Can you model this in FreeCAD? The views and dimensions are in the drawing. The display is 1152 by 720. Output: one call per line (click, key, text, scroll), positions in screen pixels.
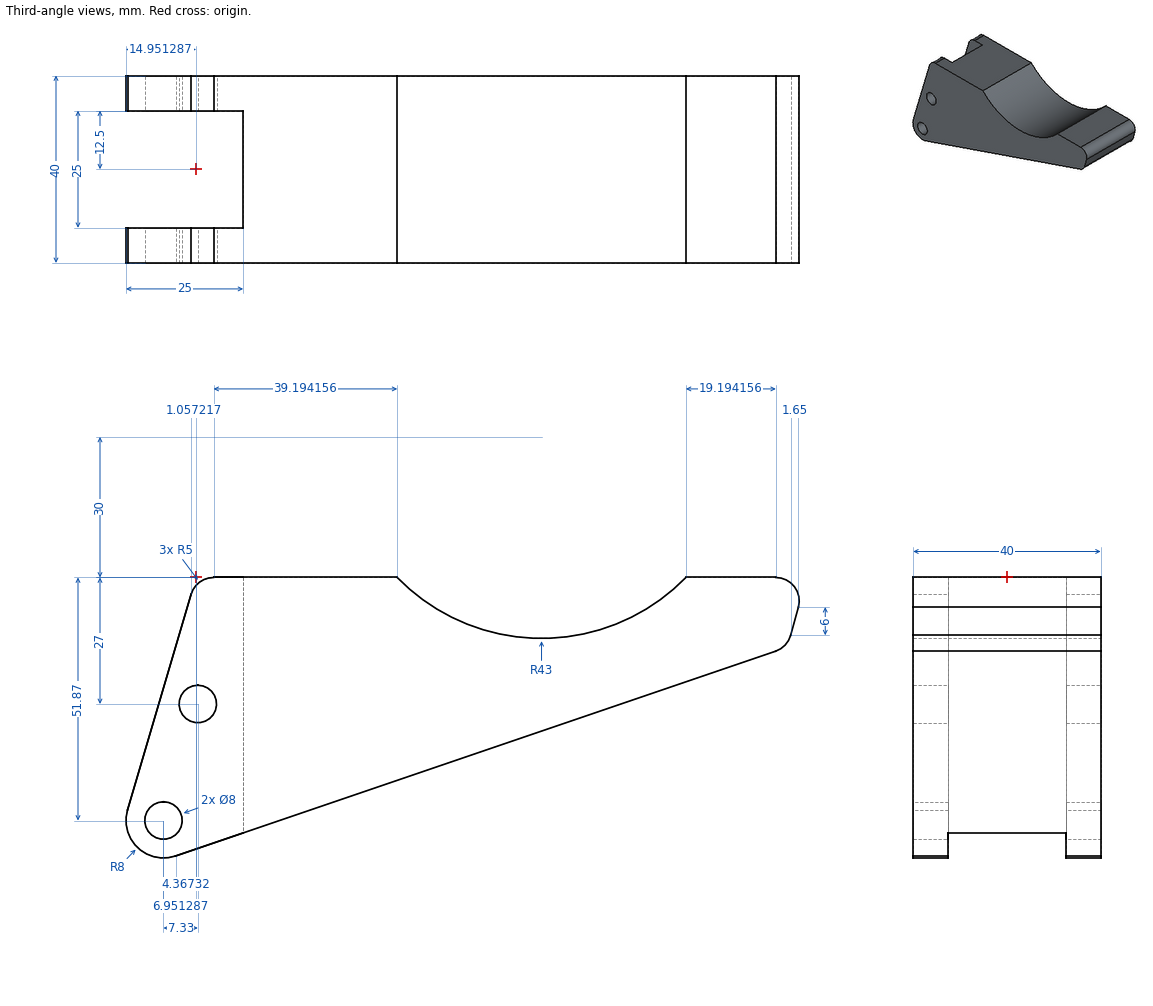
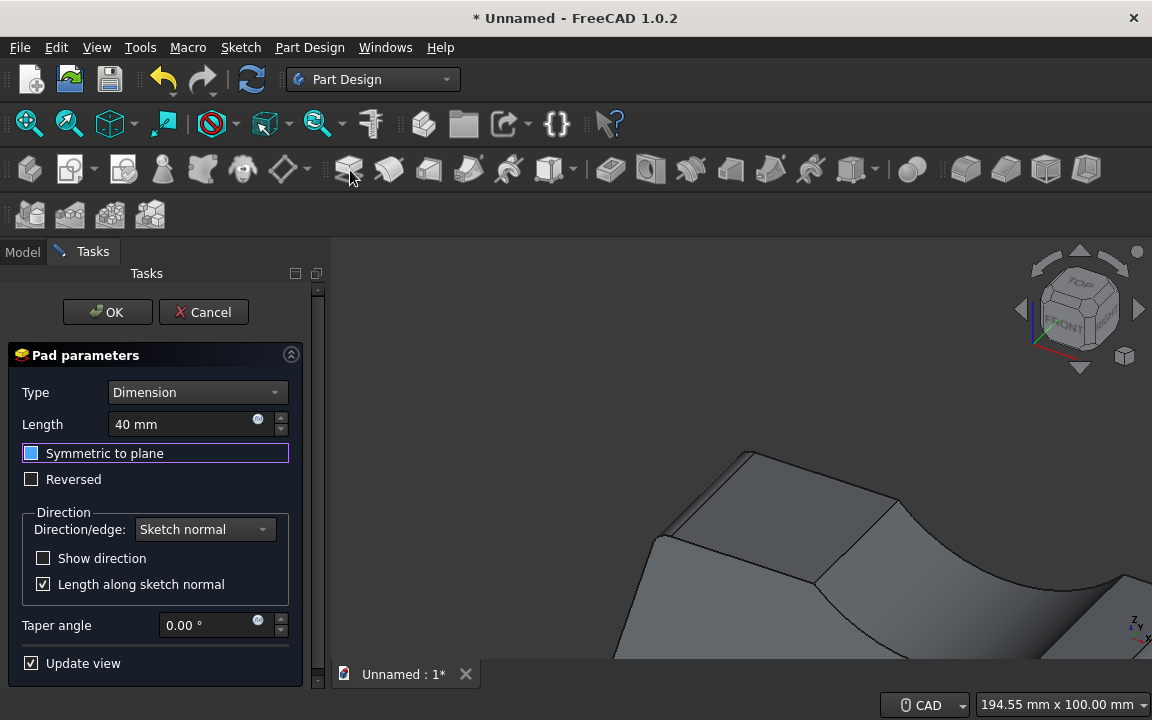
click(30, 453)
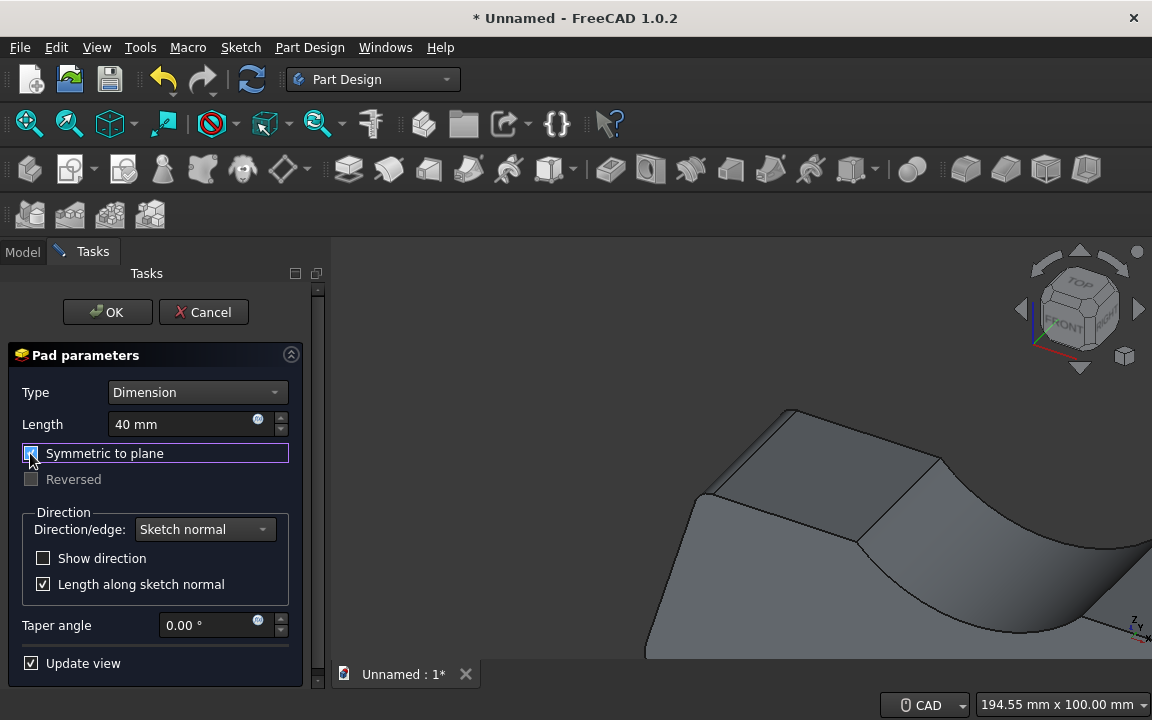
click(108, 312)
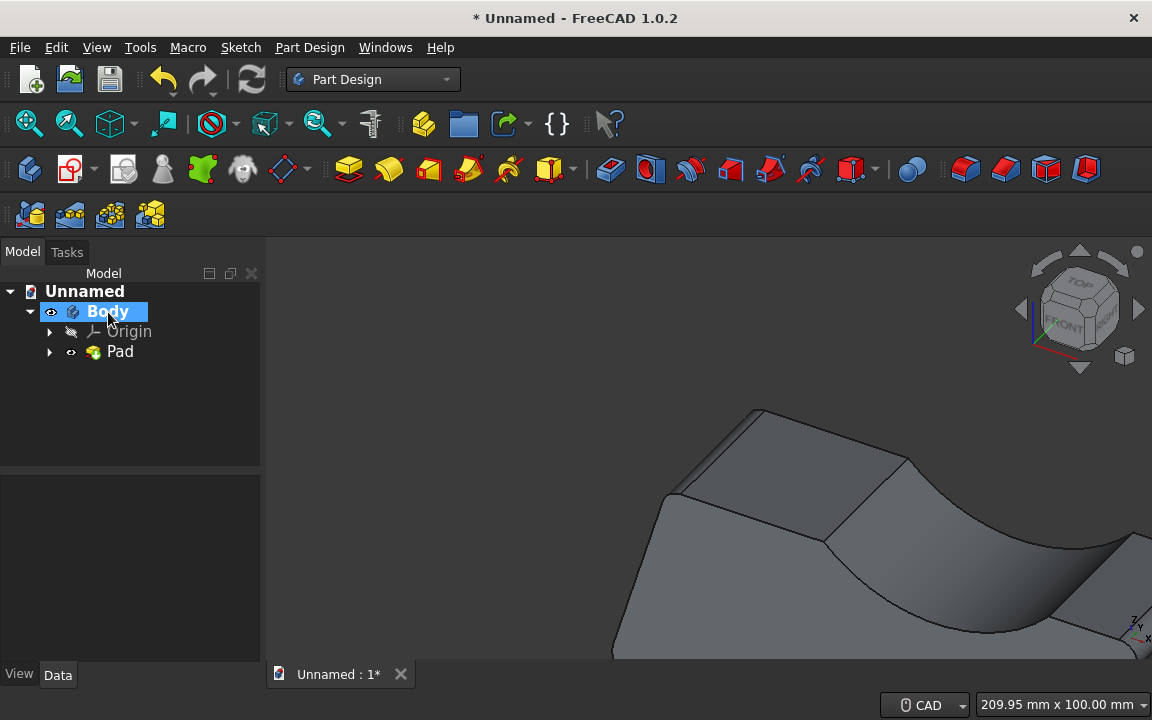
click(30, 124)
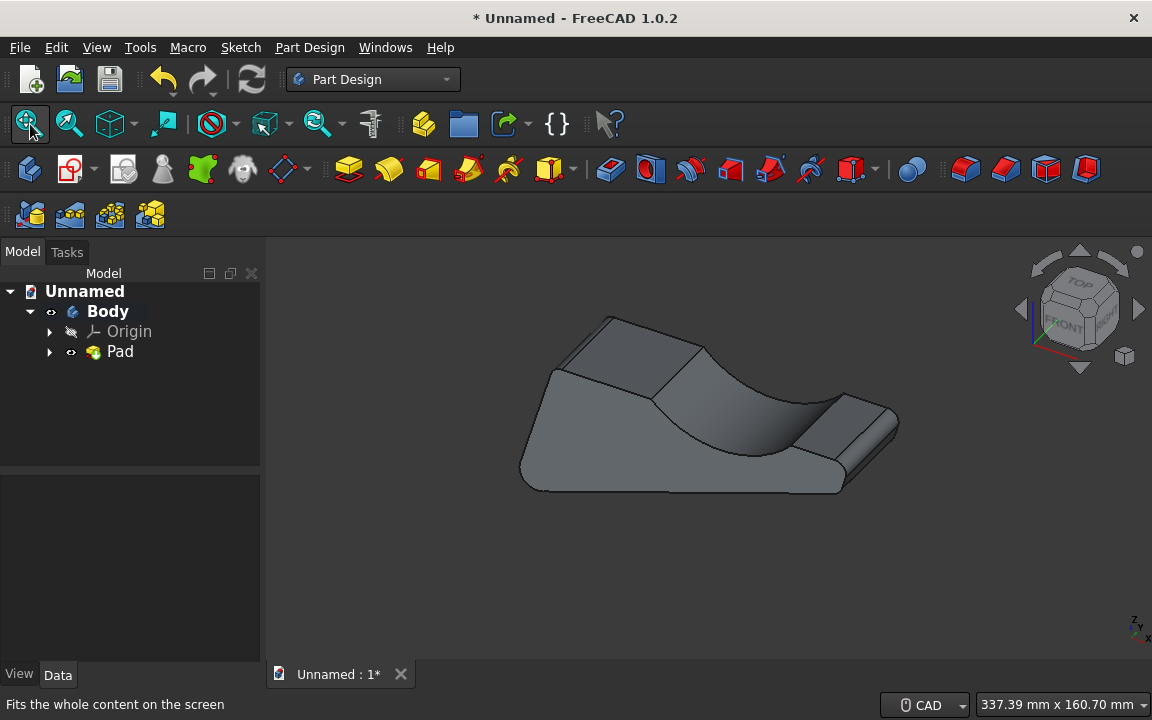
click(70, 170)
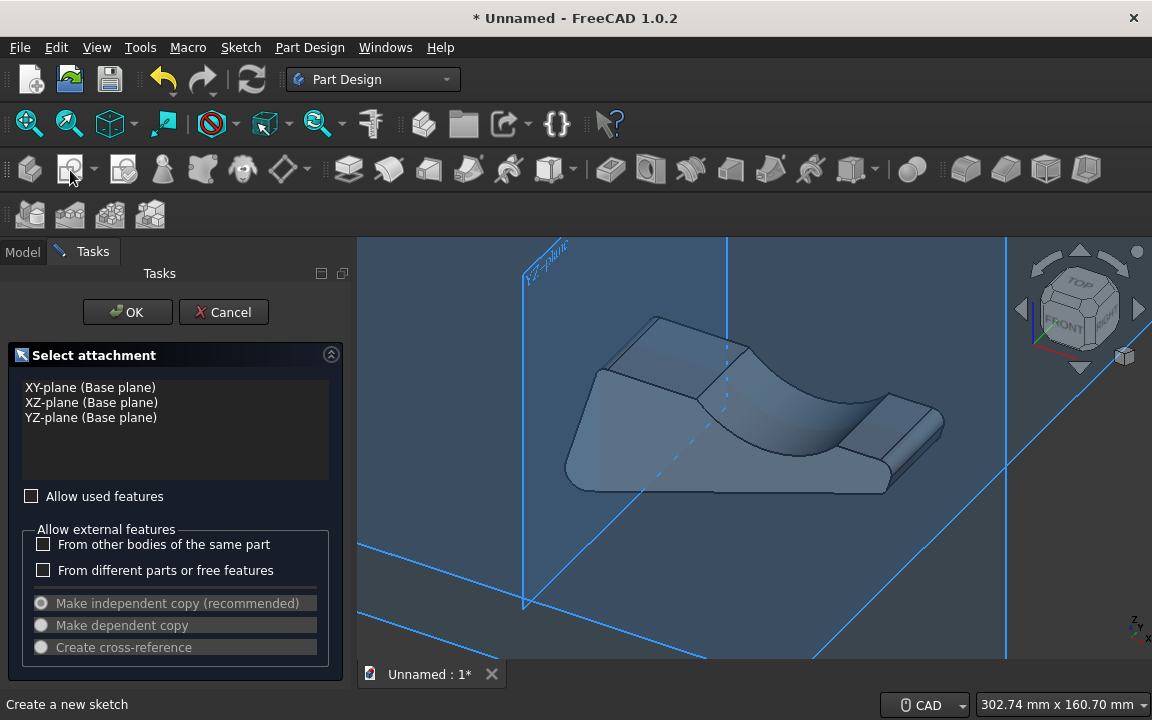
click(82, 402)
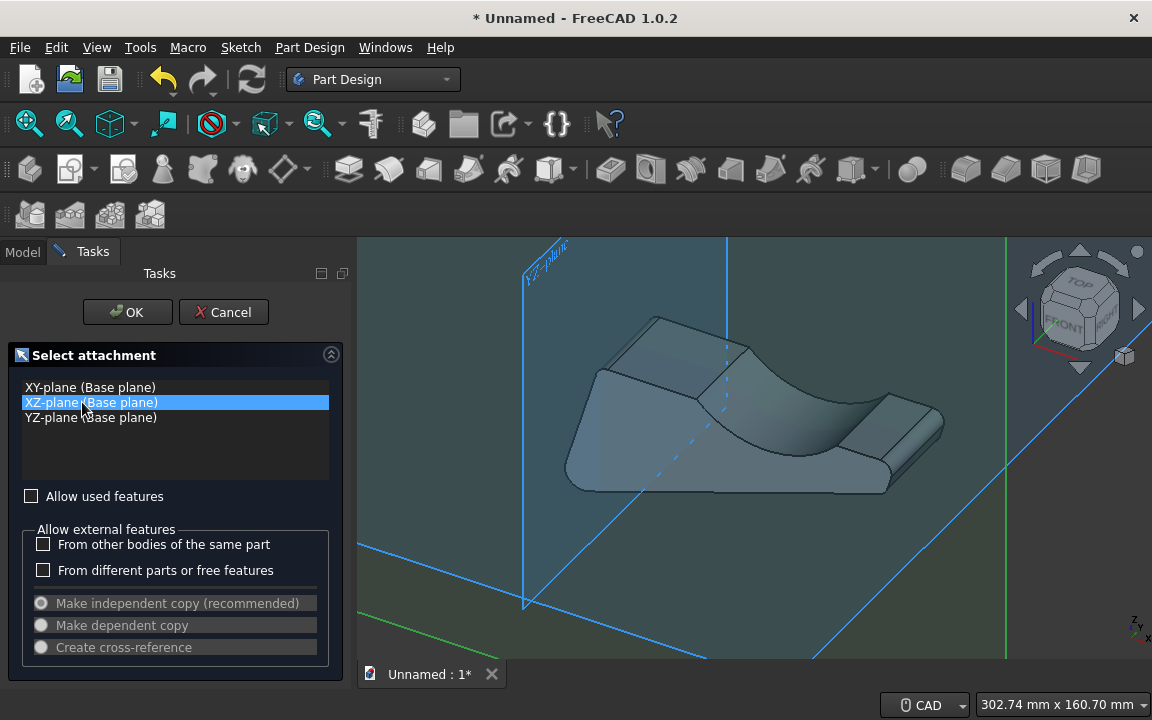
click(128, 312)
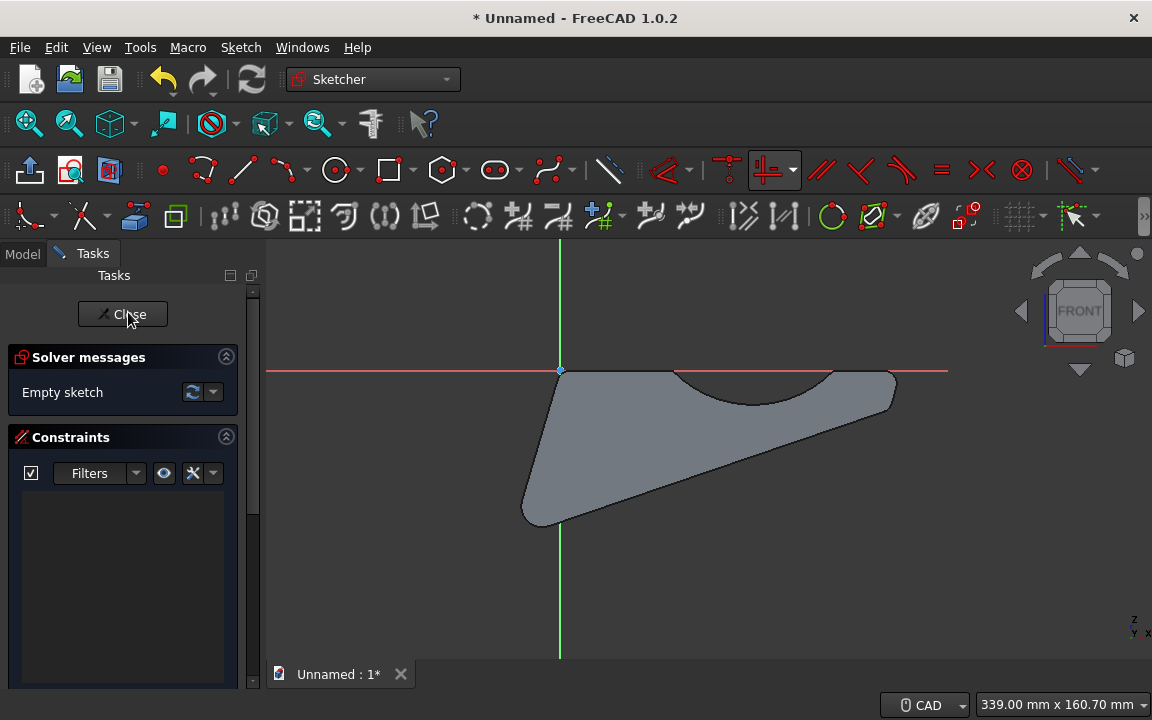
click(110, 170)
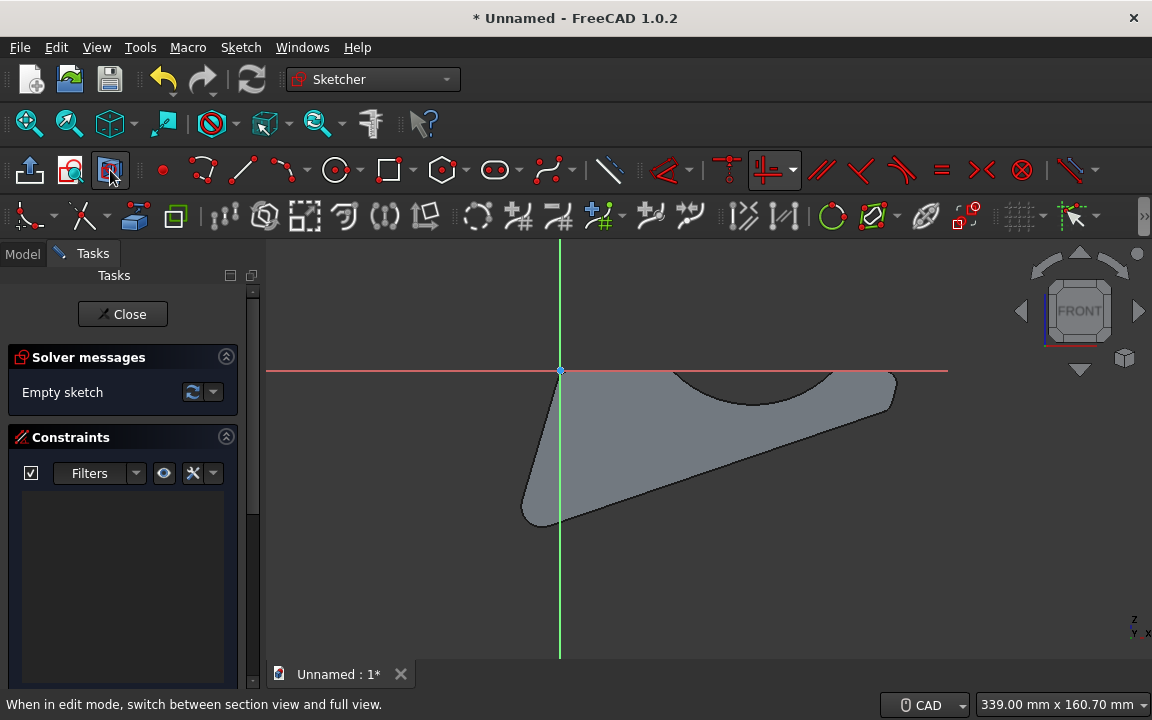
scroll(444, 438, up, 3)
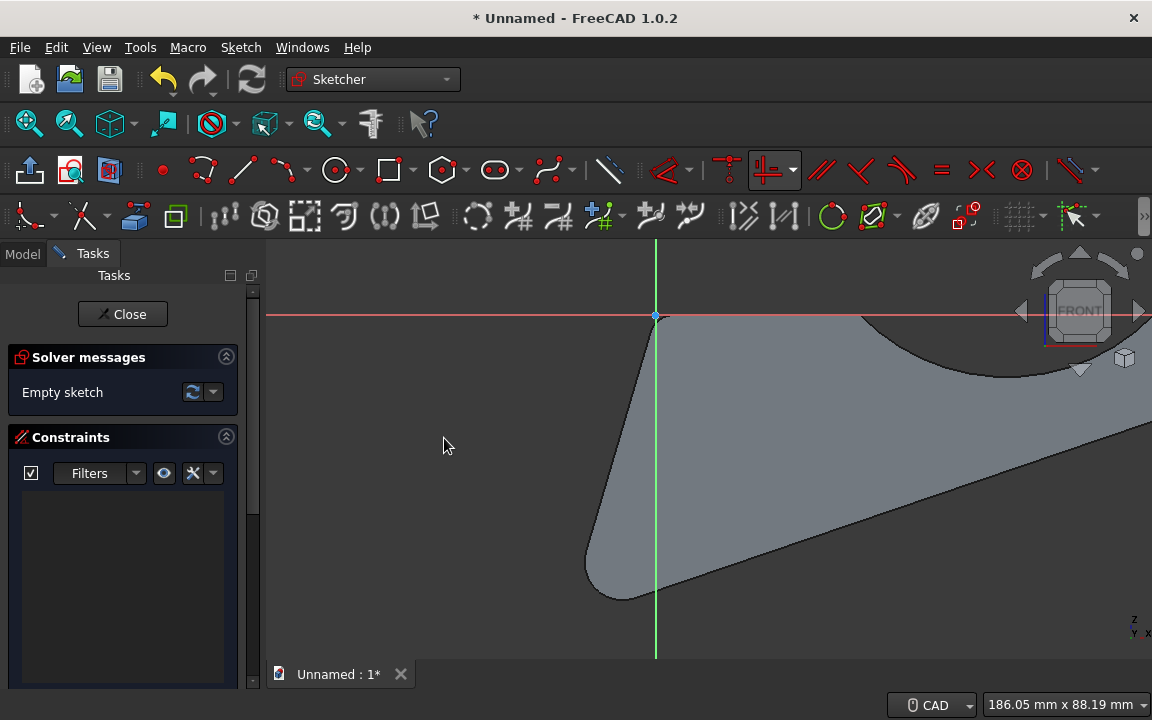
click(336, 170)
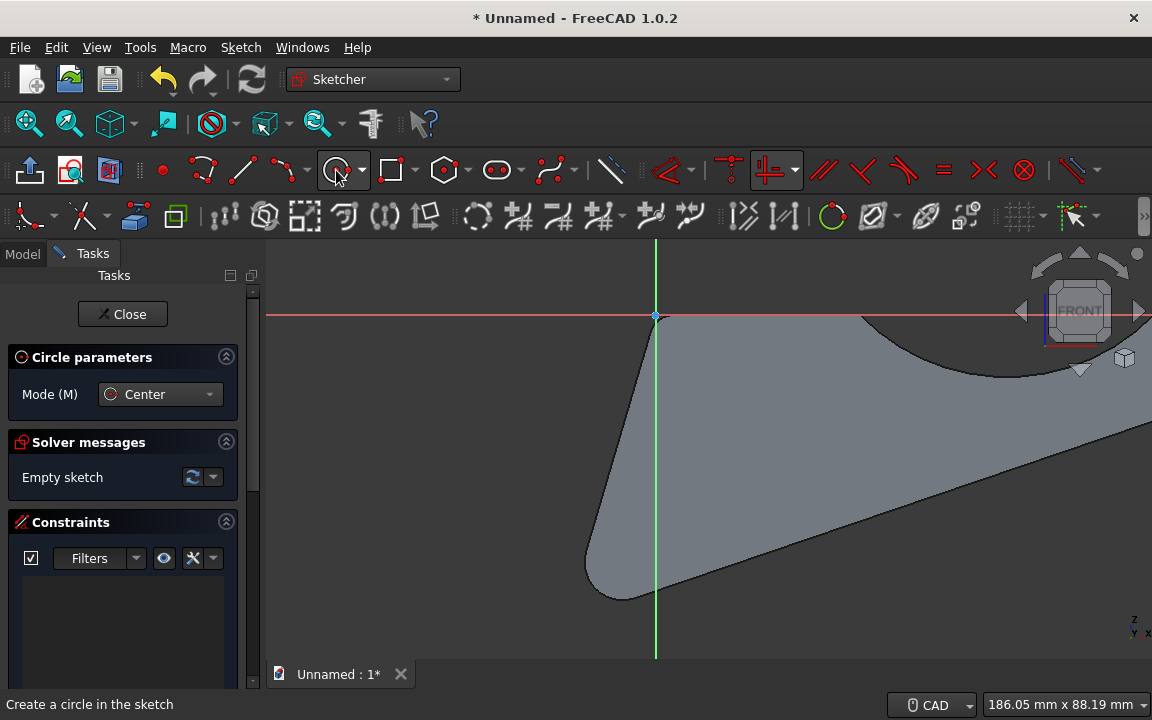
click(623, 562)
click(636, 549)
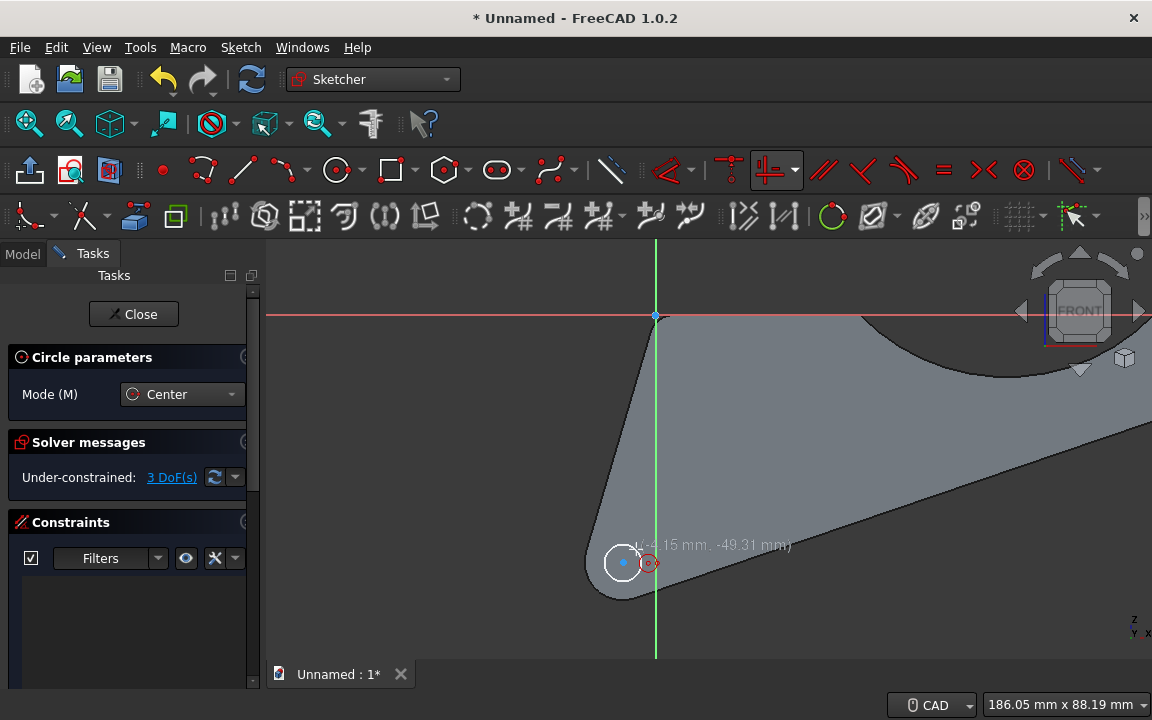
scroll(658, 444, up, 11)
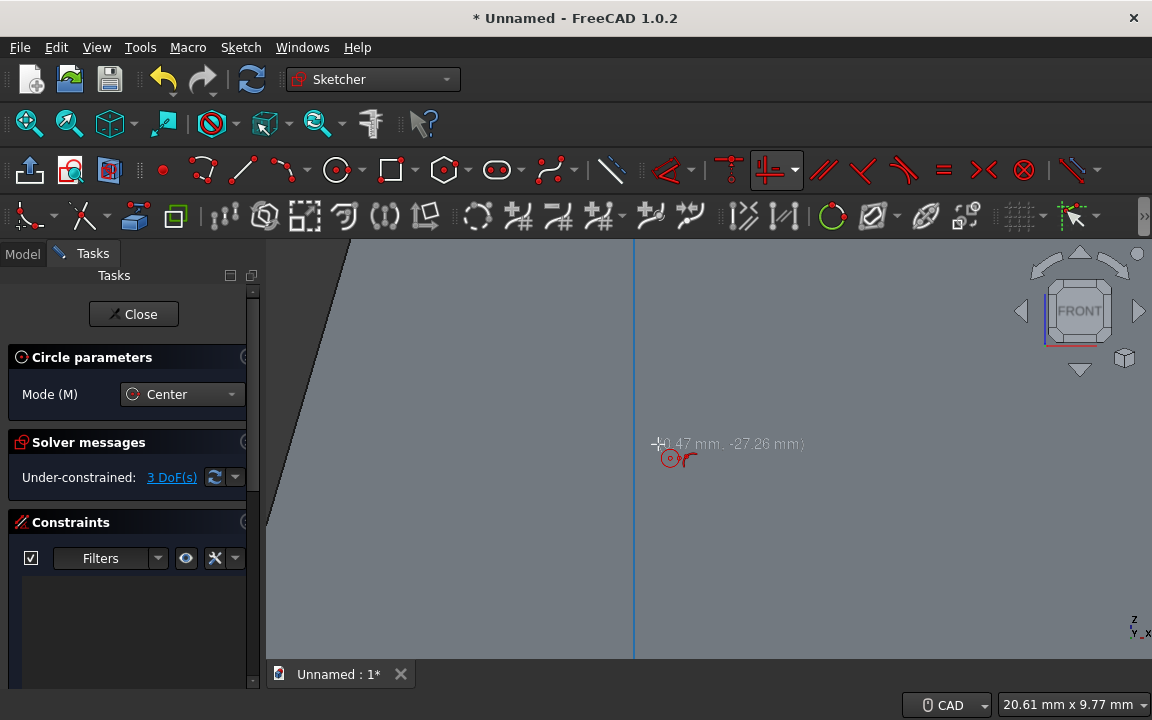
click(650, 438)